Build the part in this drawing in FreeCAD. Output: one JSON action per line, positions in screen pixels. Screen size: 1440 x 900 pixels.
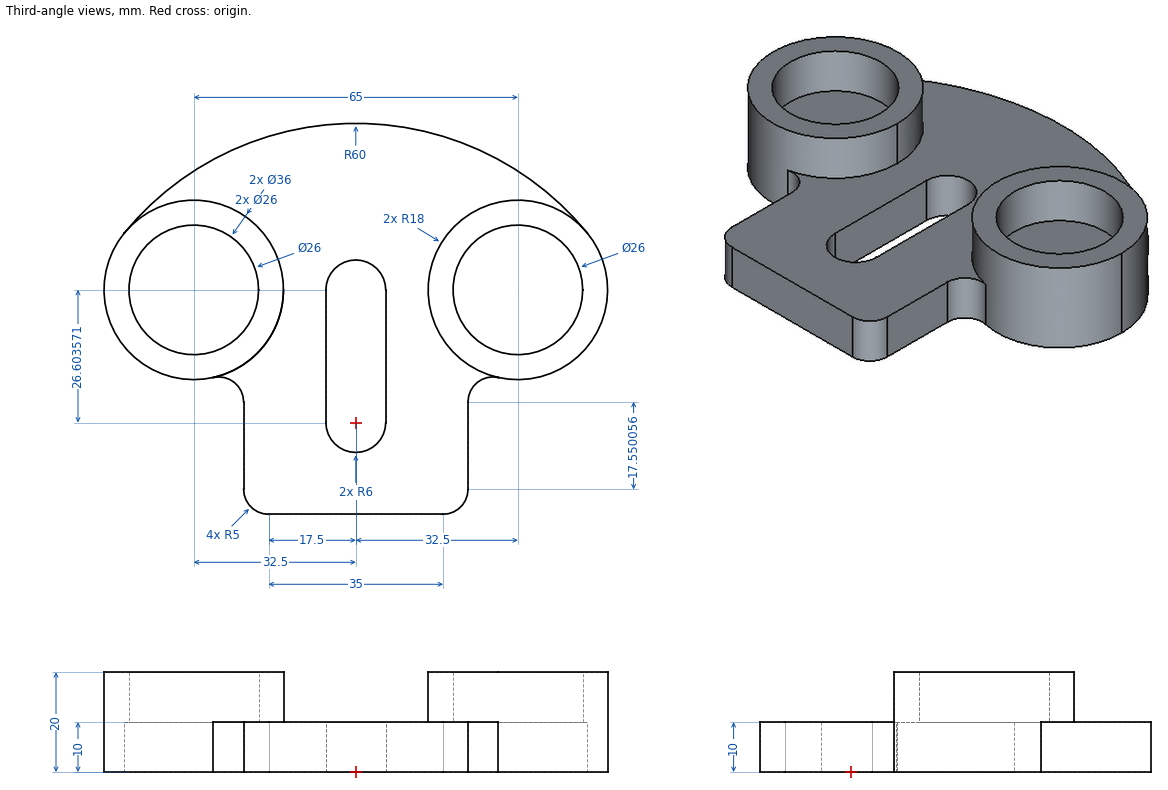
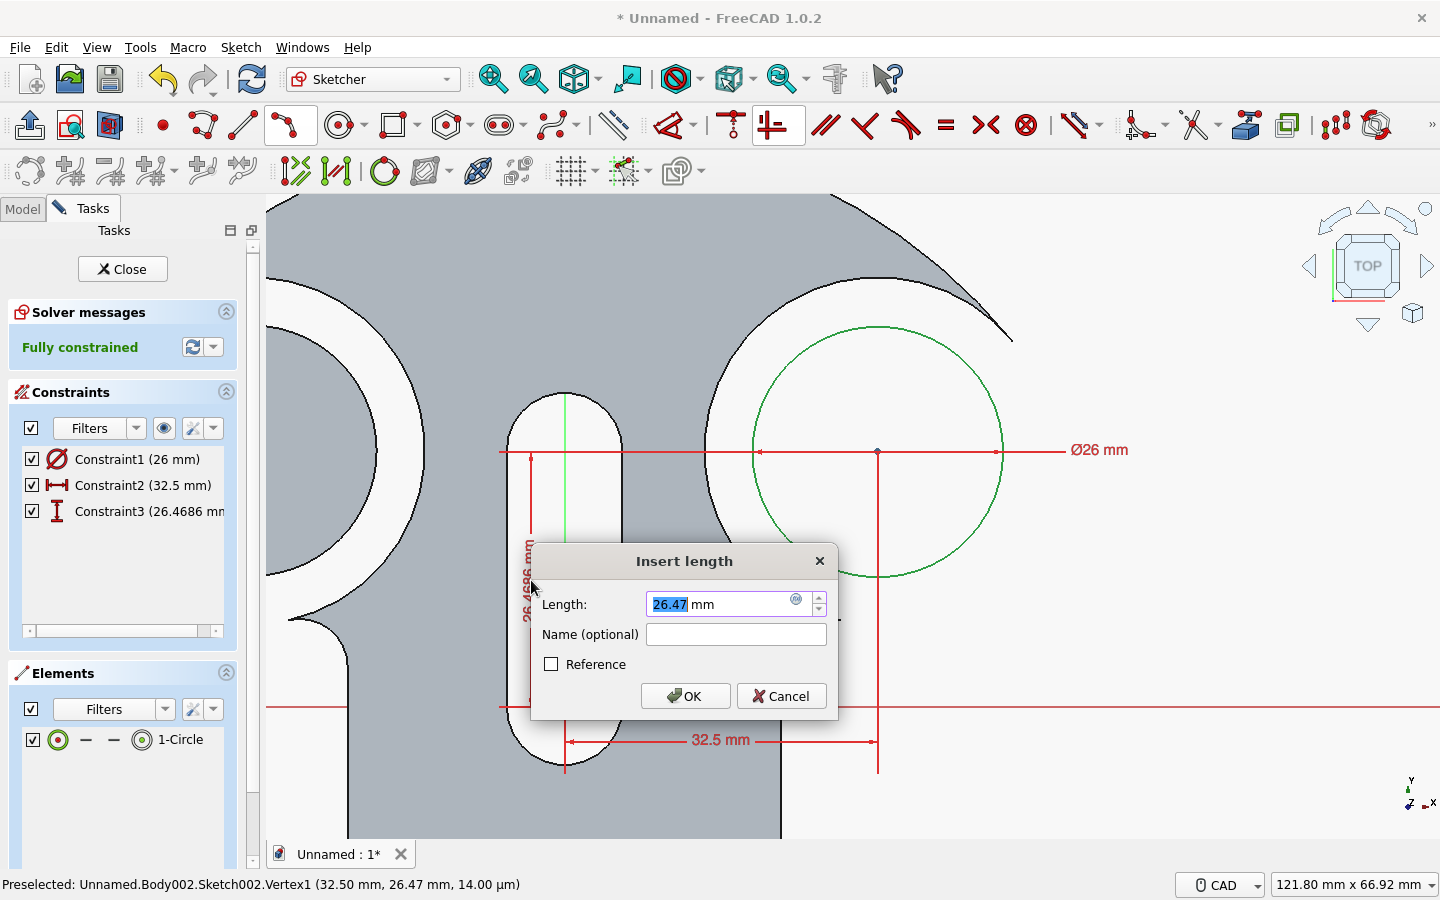
{"action": "type", "text": "26.603571"}
{"action": "key", "text": "Return"}
{"action": "key", "text": "Escape"}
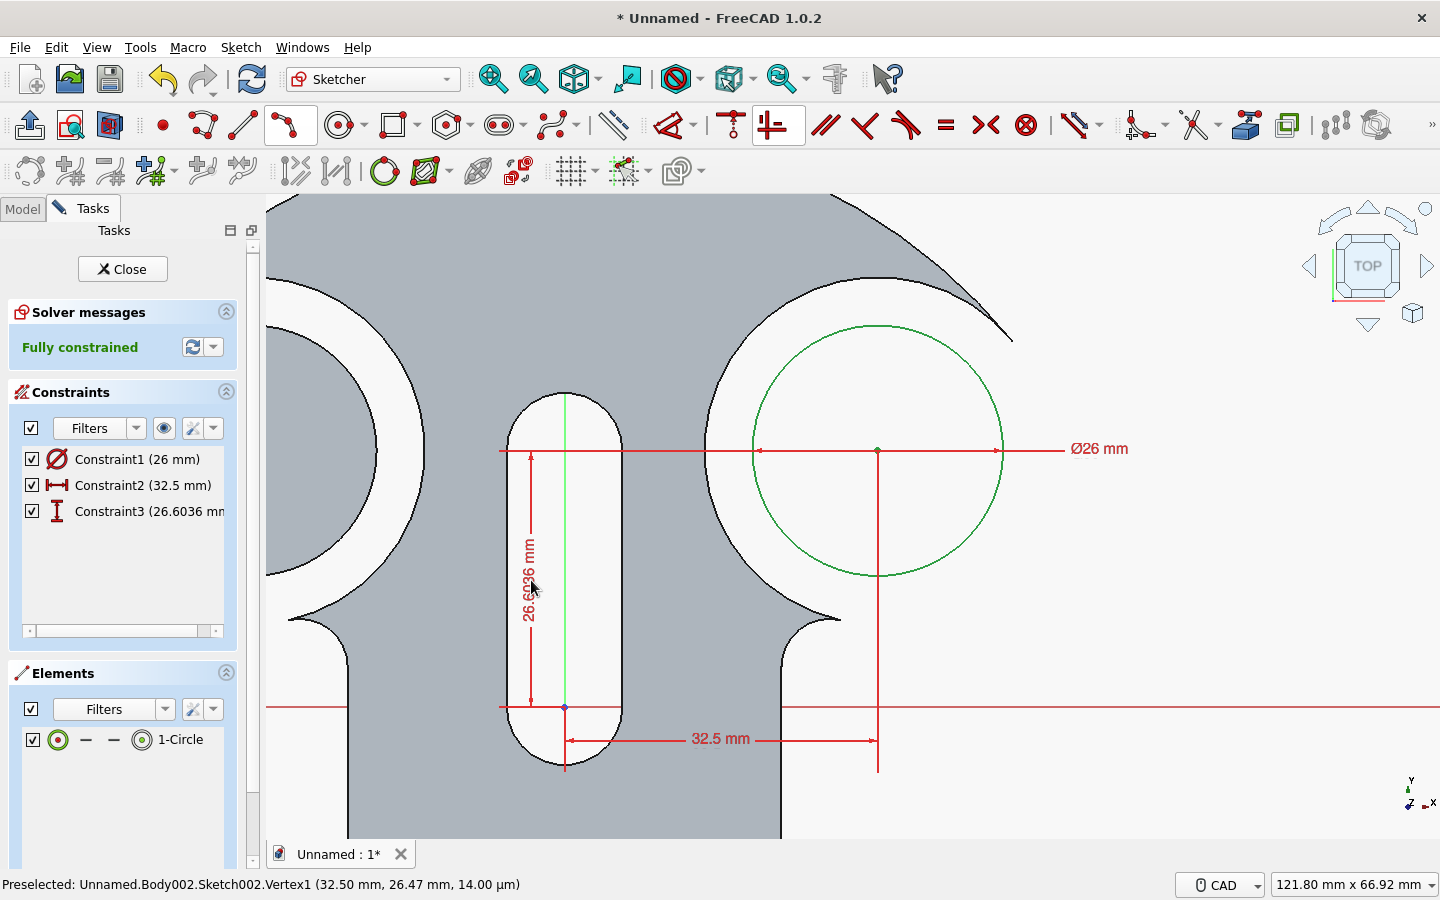
{"action": "left_click", "coordinate": [123, 269]}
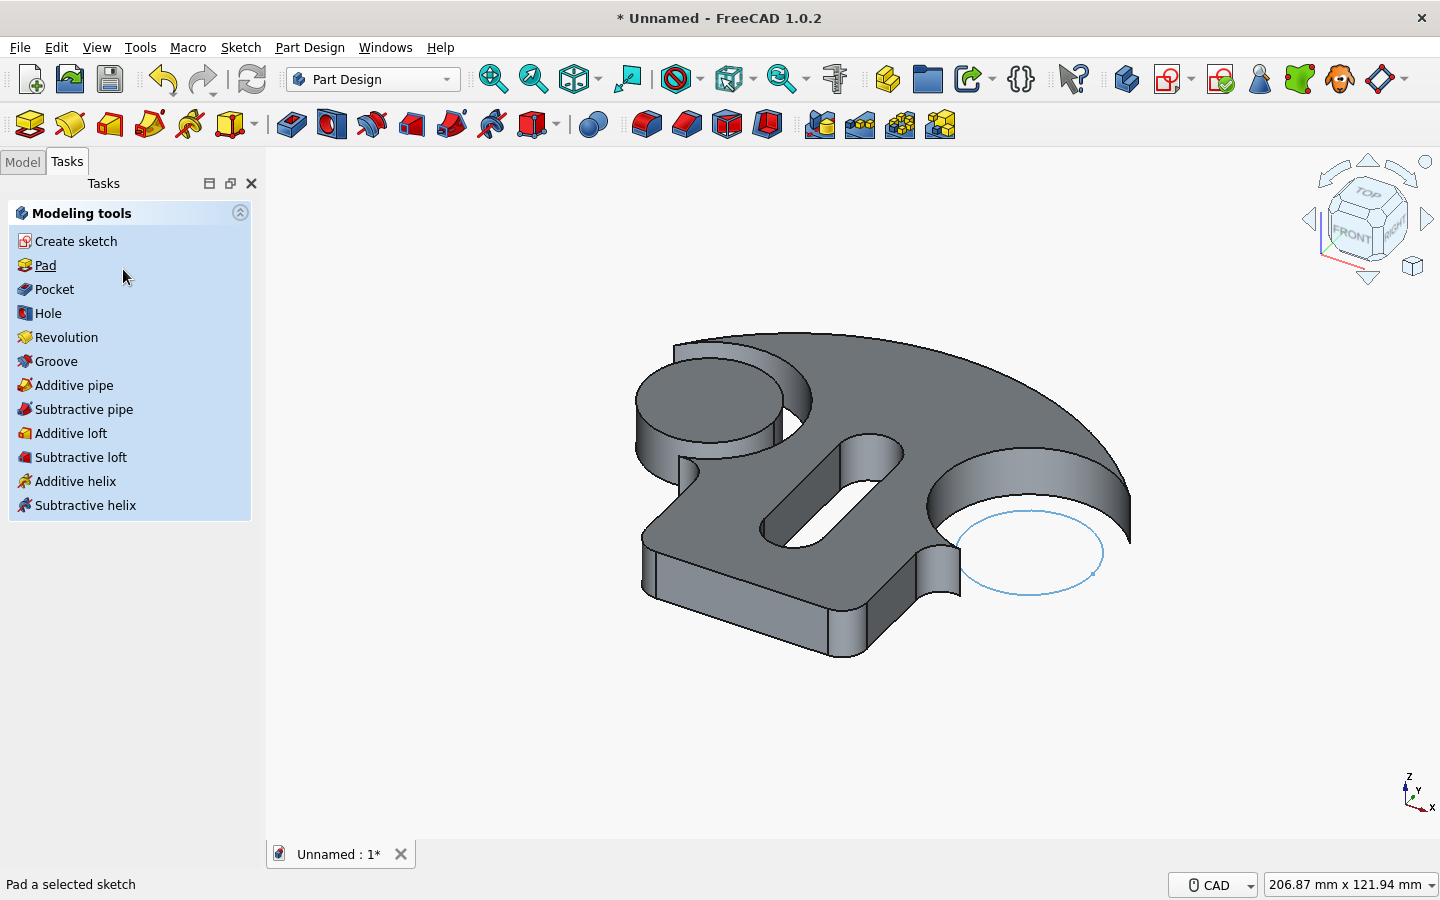
{"action": "left_click", "coordinate": [30, 124]}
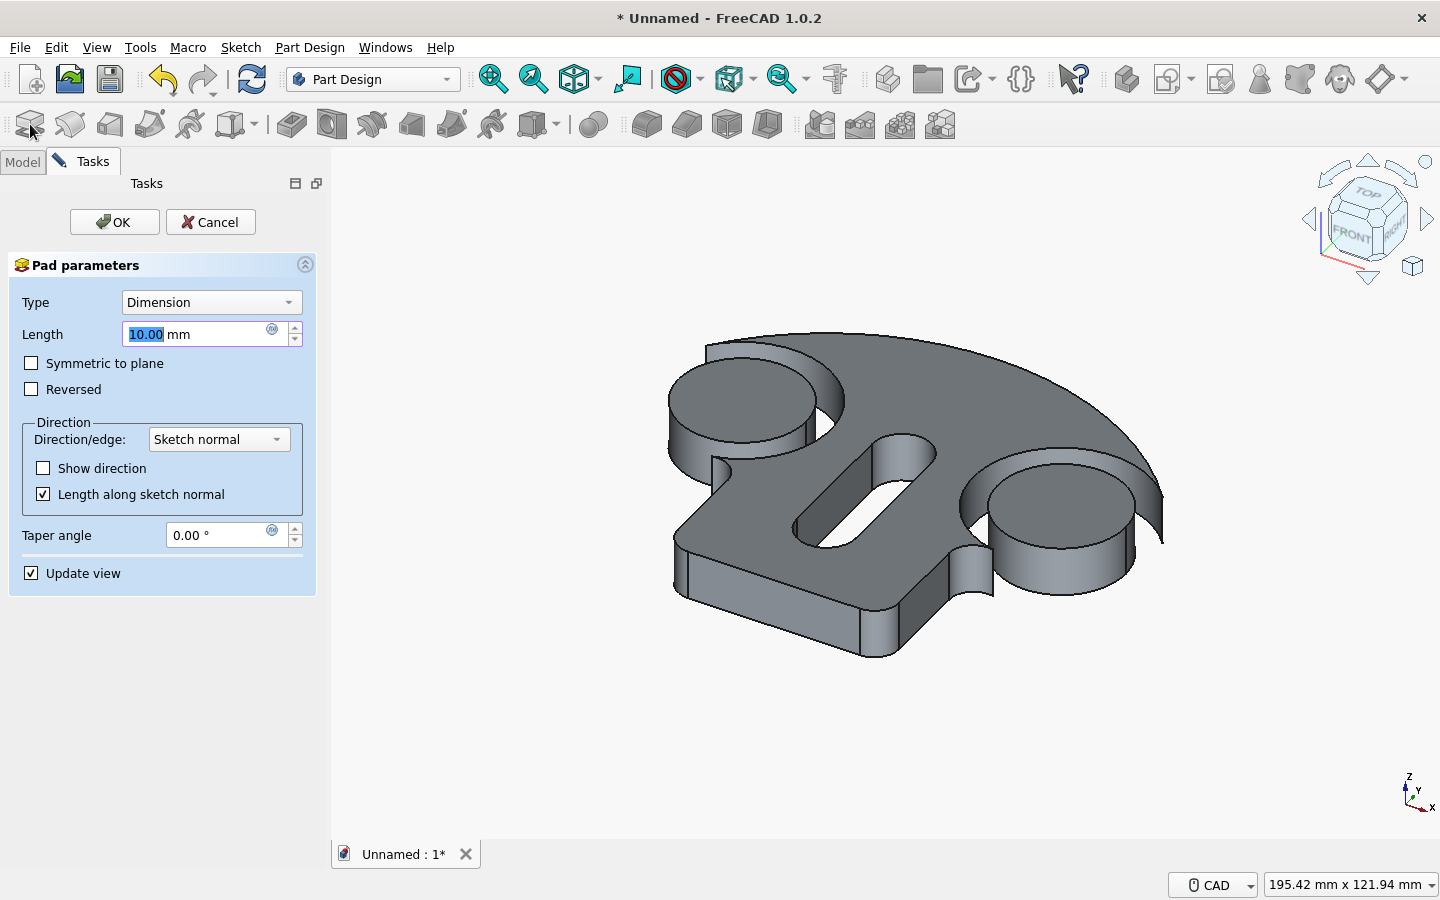
{"action": "type", "text": "10"}
{"action": "key", "text": "Tab"}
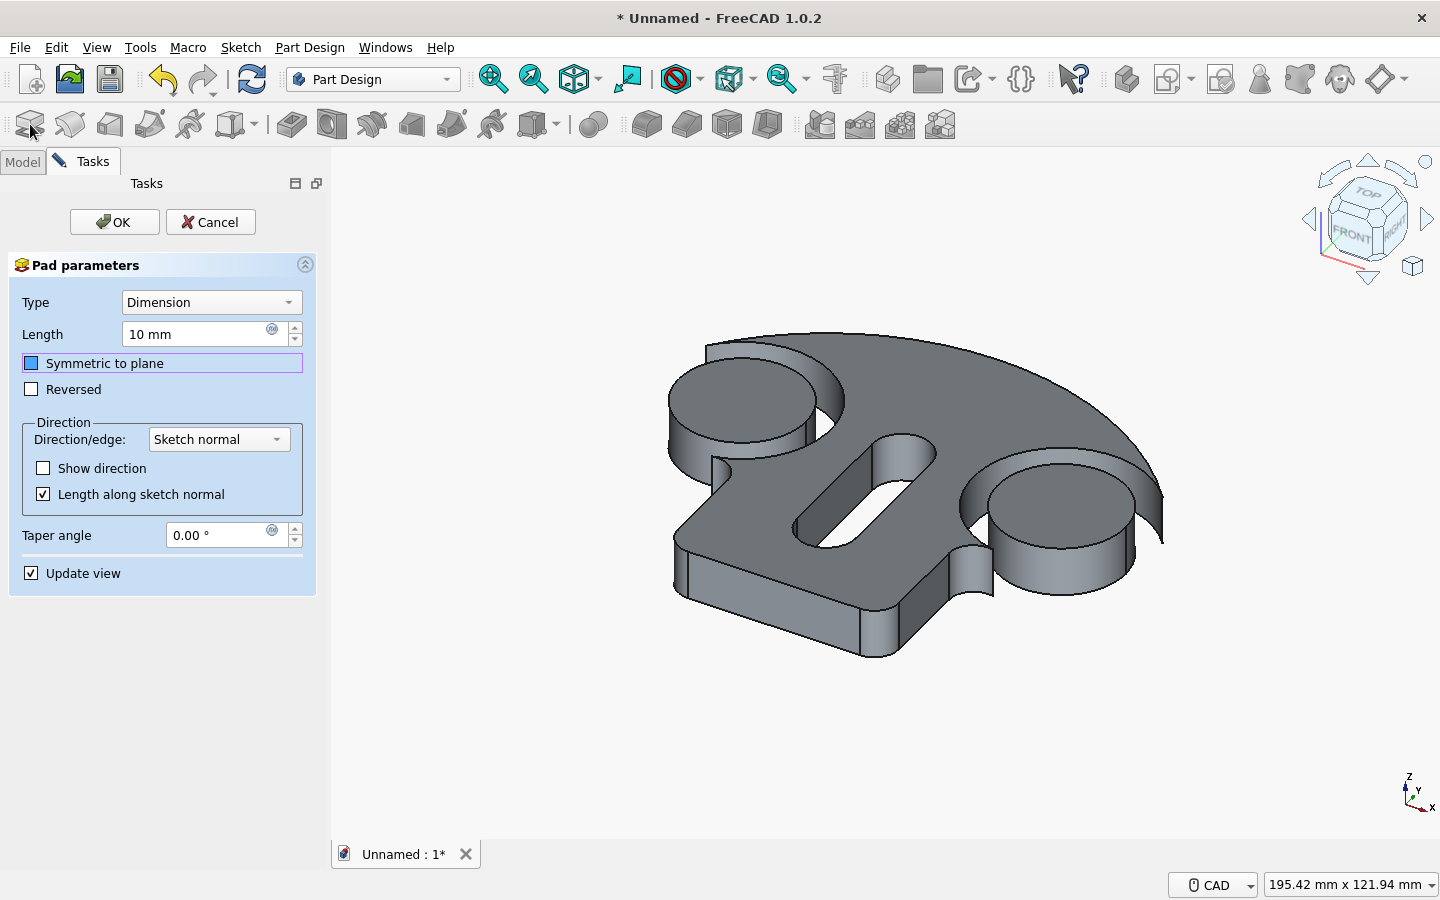
{"action": "left_click", "coordinate": [115, 222]}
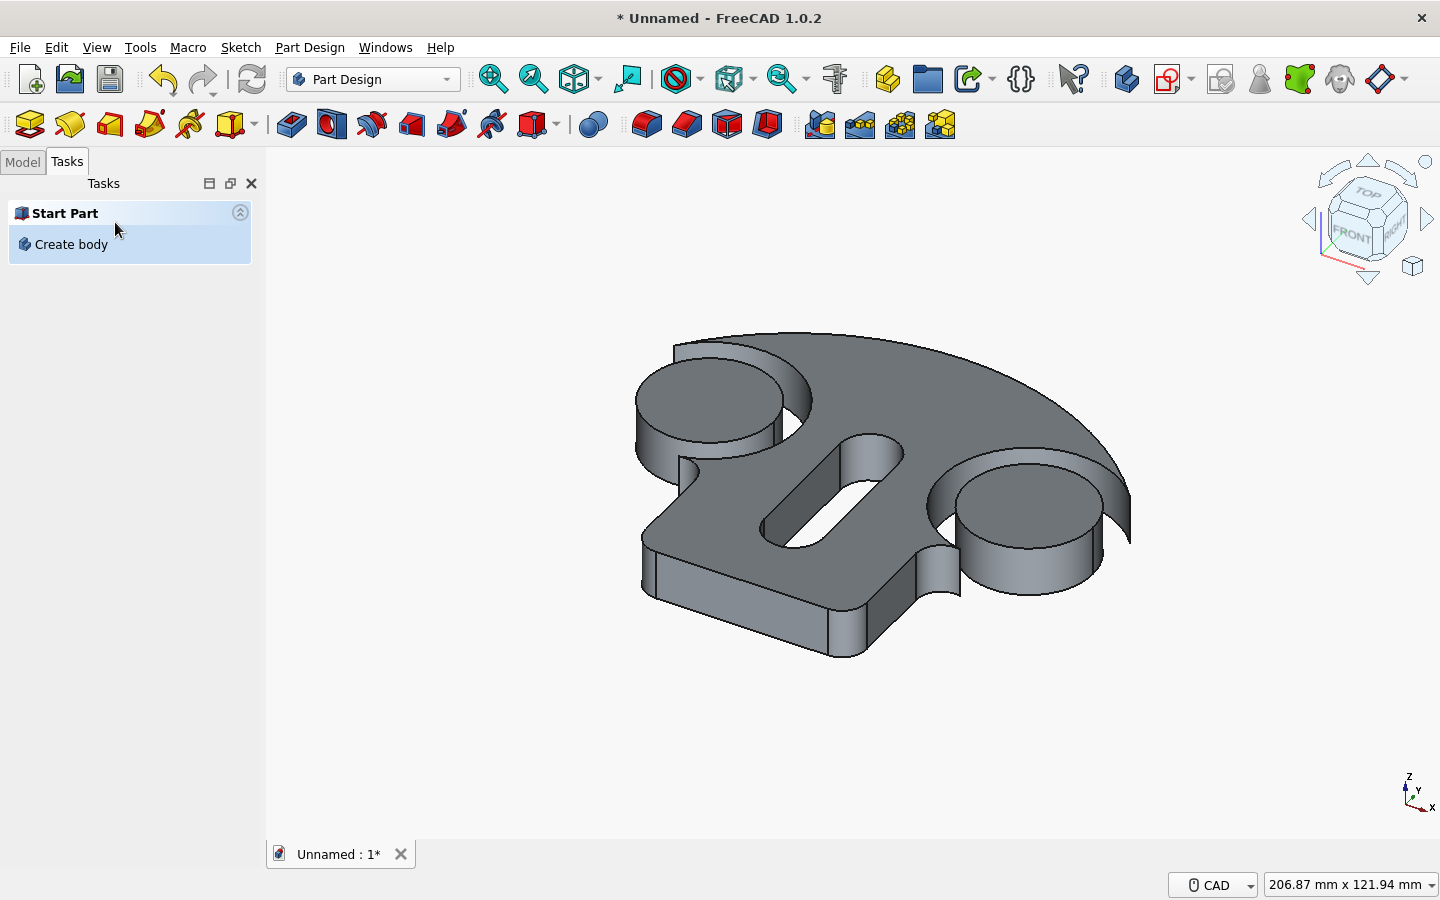
{"action": "left_click", "coordinate": [494, 80]}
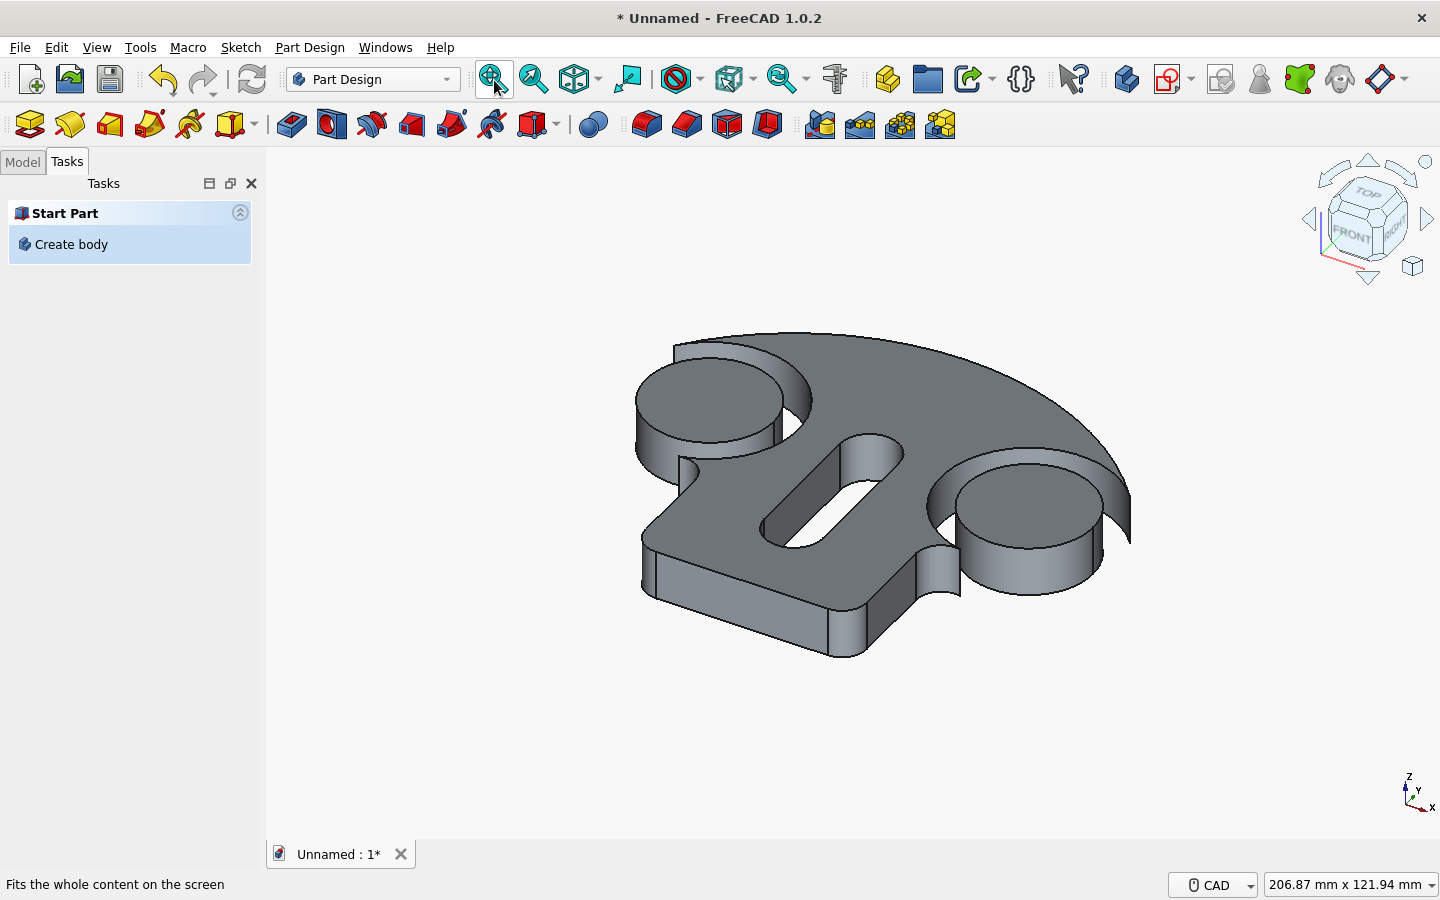
{"action": "left_click", "coordinate": [23, 161]}